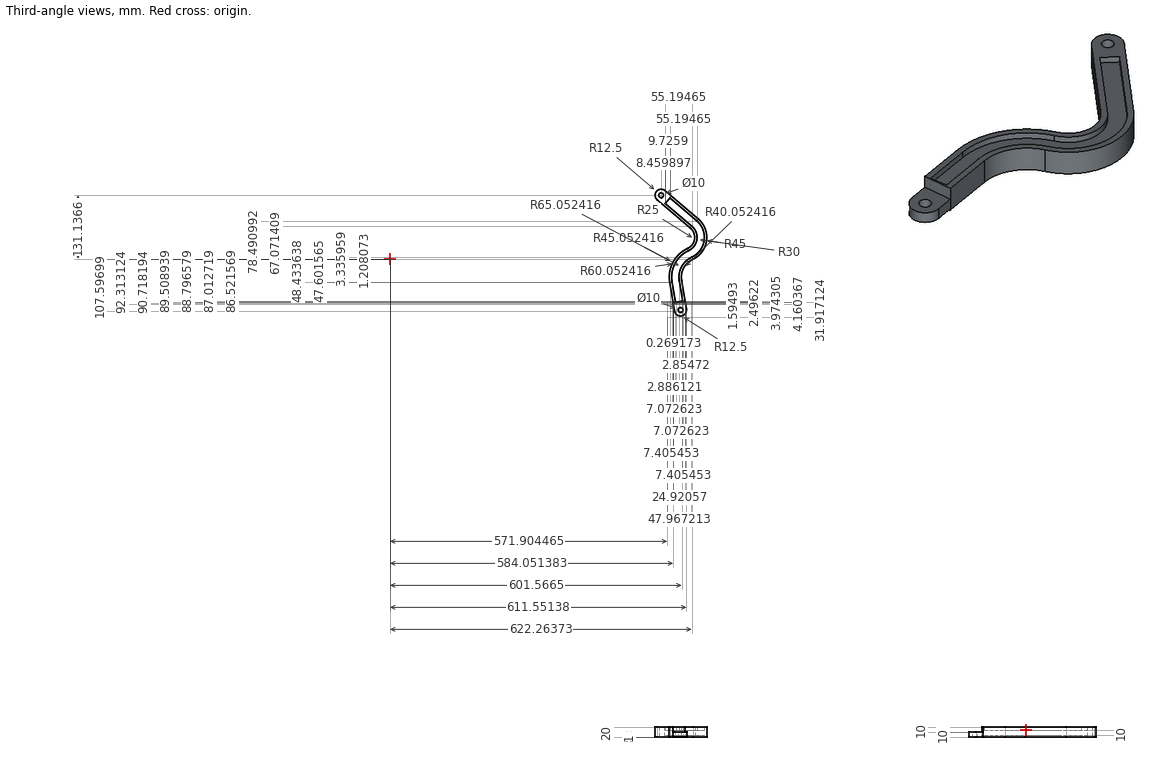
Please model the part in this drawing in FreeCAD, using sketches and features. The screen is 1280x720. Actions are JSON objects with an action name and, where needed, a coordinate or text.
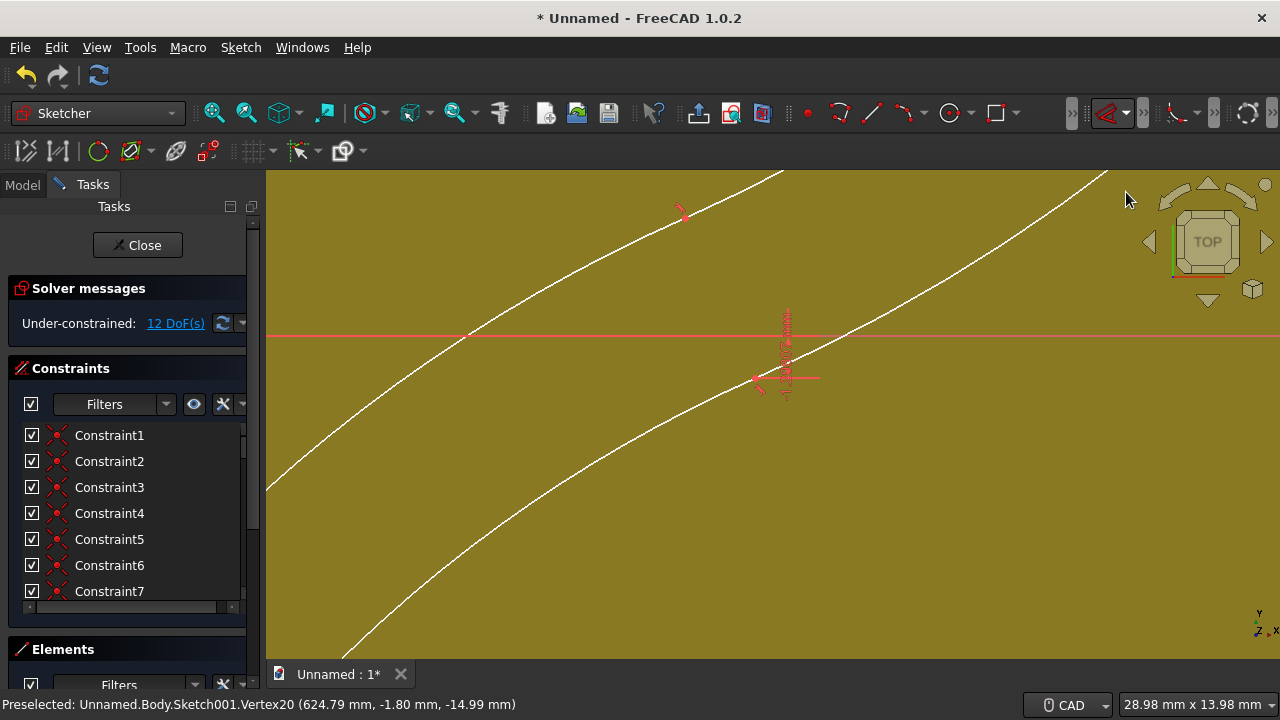
{"action": "scroll", "coordinate": [737, 454], "scroll_direction": "down", "scroll_amount": 16}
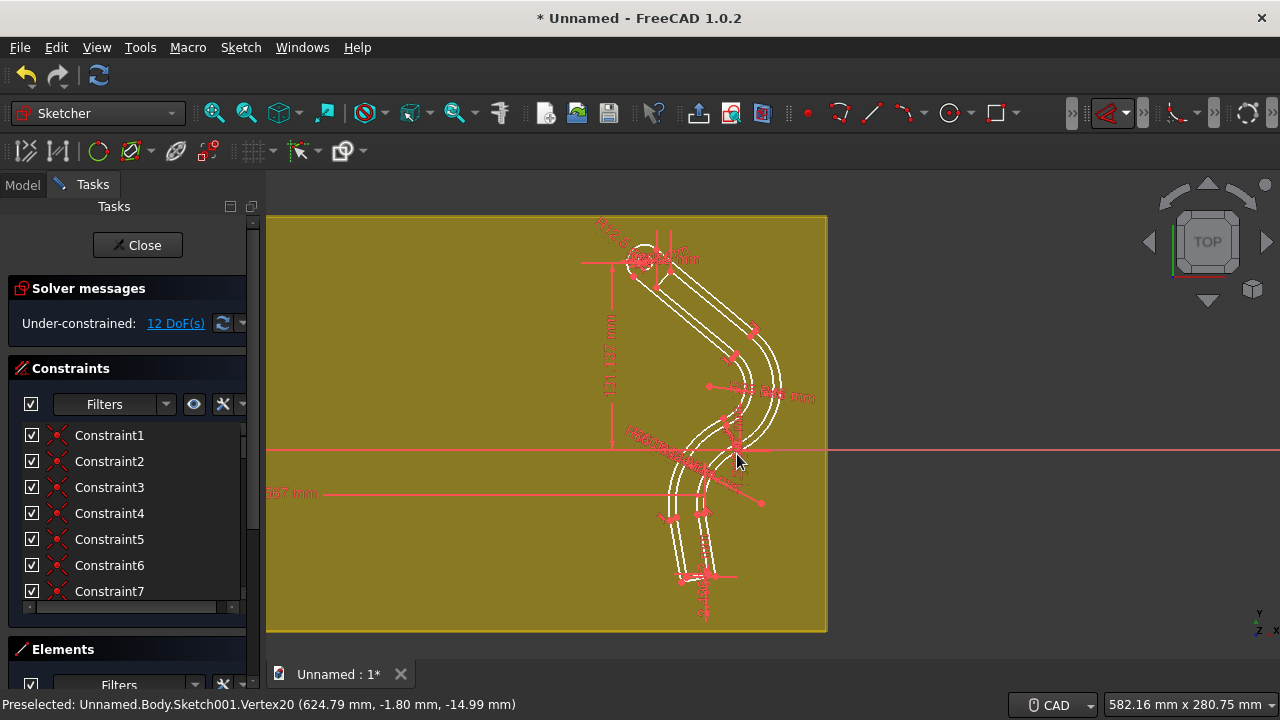
{"action": "scroll", "coordinate": [673, 539], "scroll_direction": "up", "scroll_amount": 7}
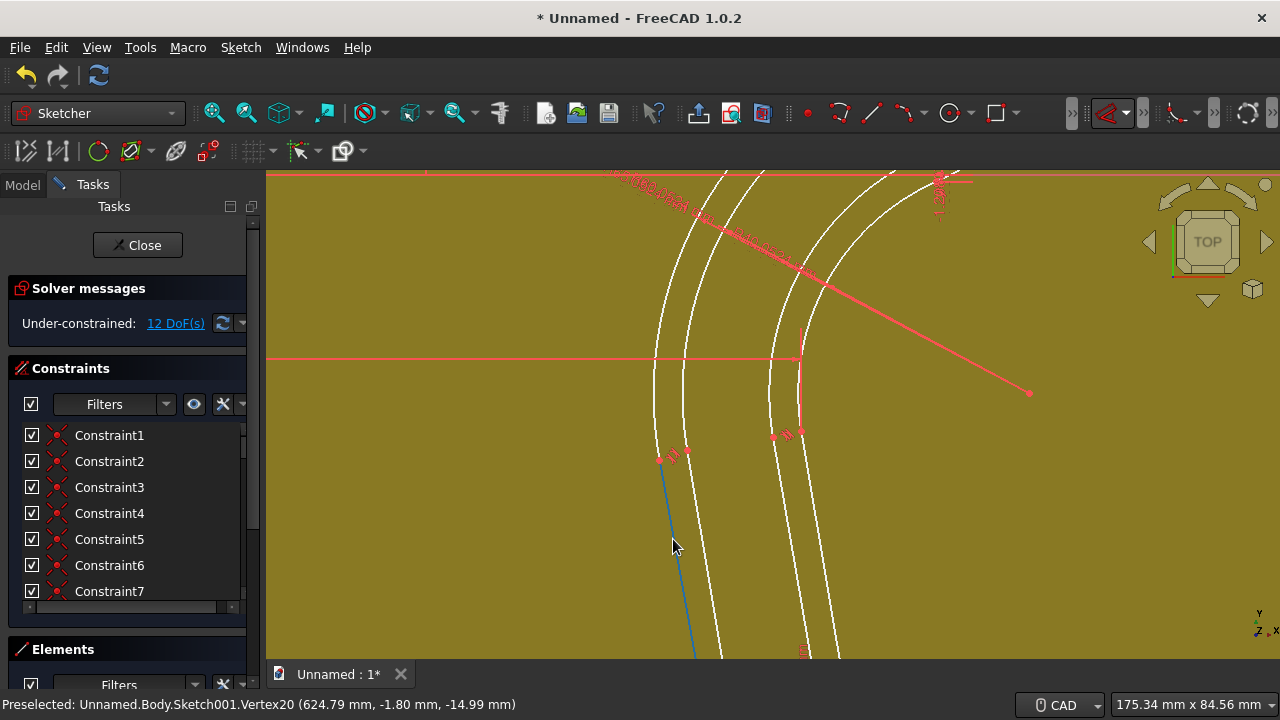
{"action": "left_click", "coordinate": [673, 536]}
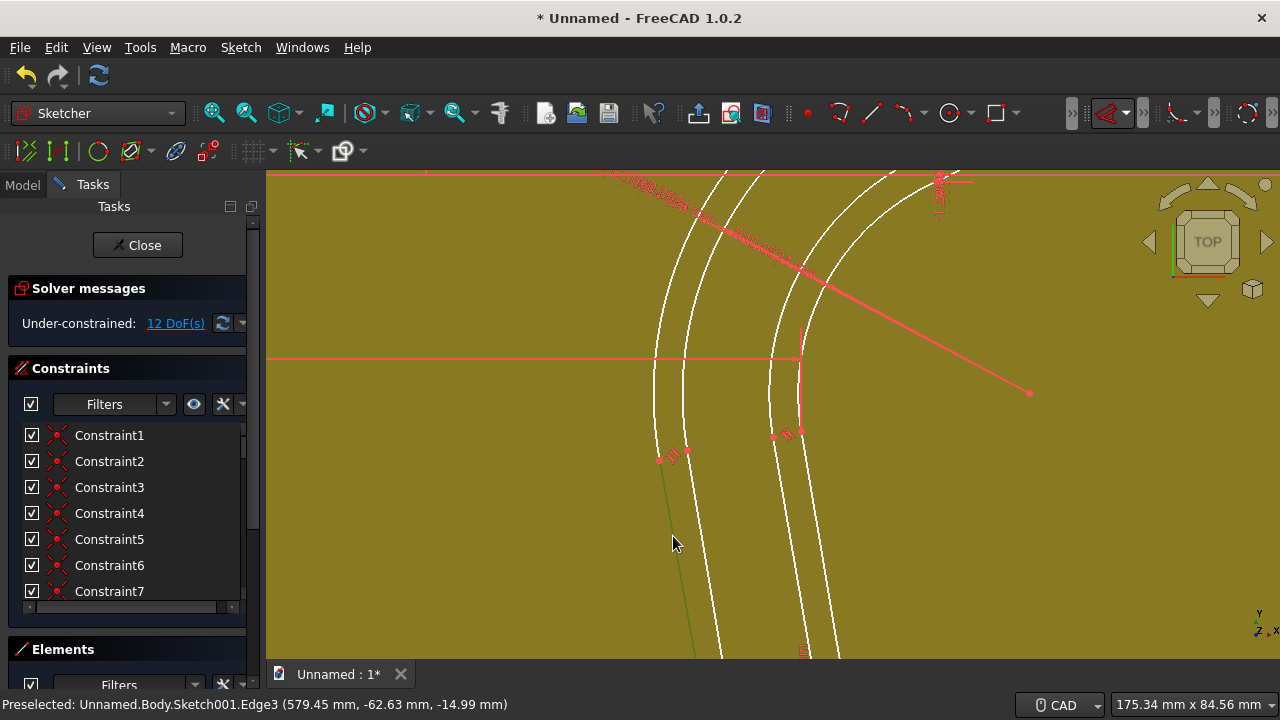
{"action": "left_click", "coordinate": [1128, 114]}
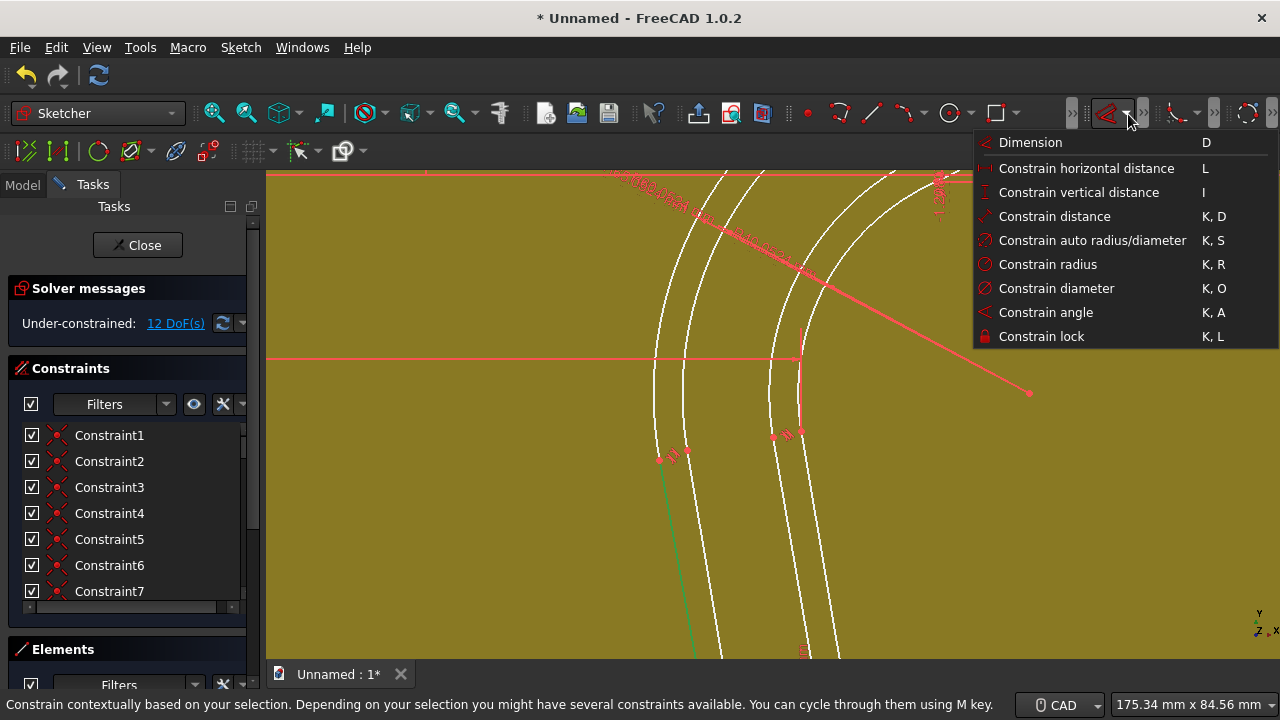
{"action": "left_click", "coordinate": [1126, 168]}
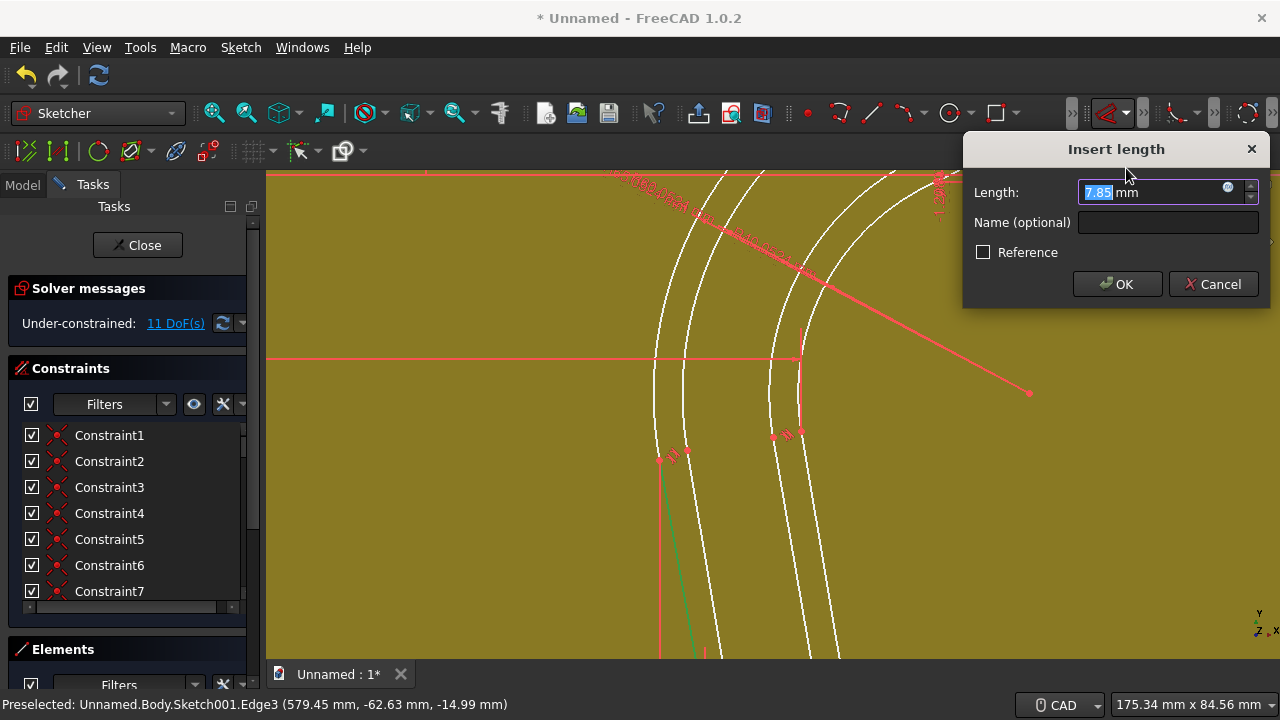
{"action": "type", "text": "7.405453"}
{"action": "key", "text": "Return"}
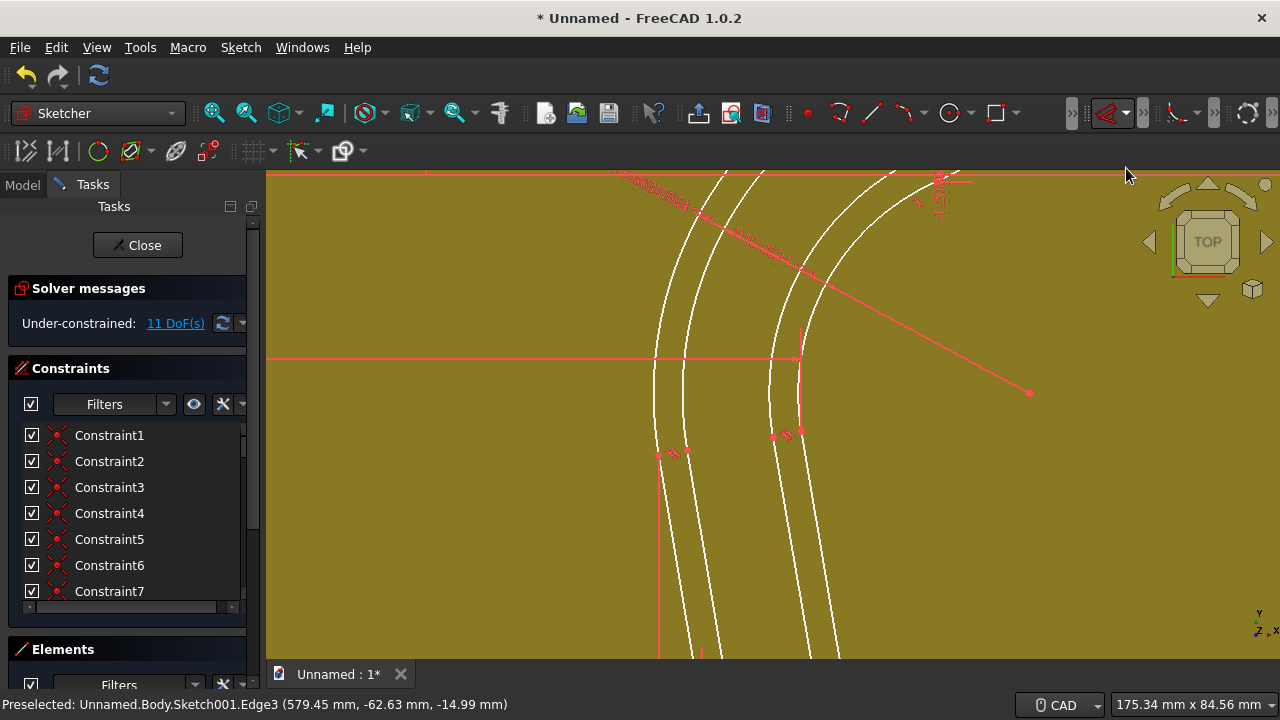
{"action": "scroll", "coordinate": [673, 539], "scroll_direction": "down", "scroll_amount": 7}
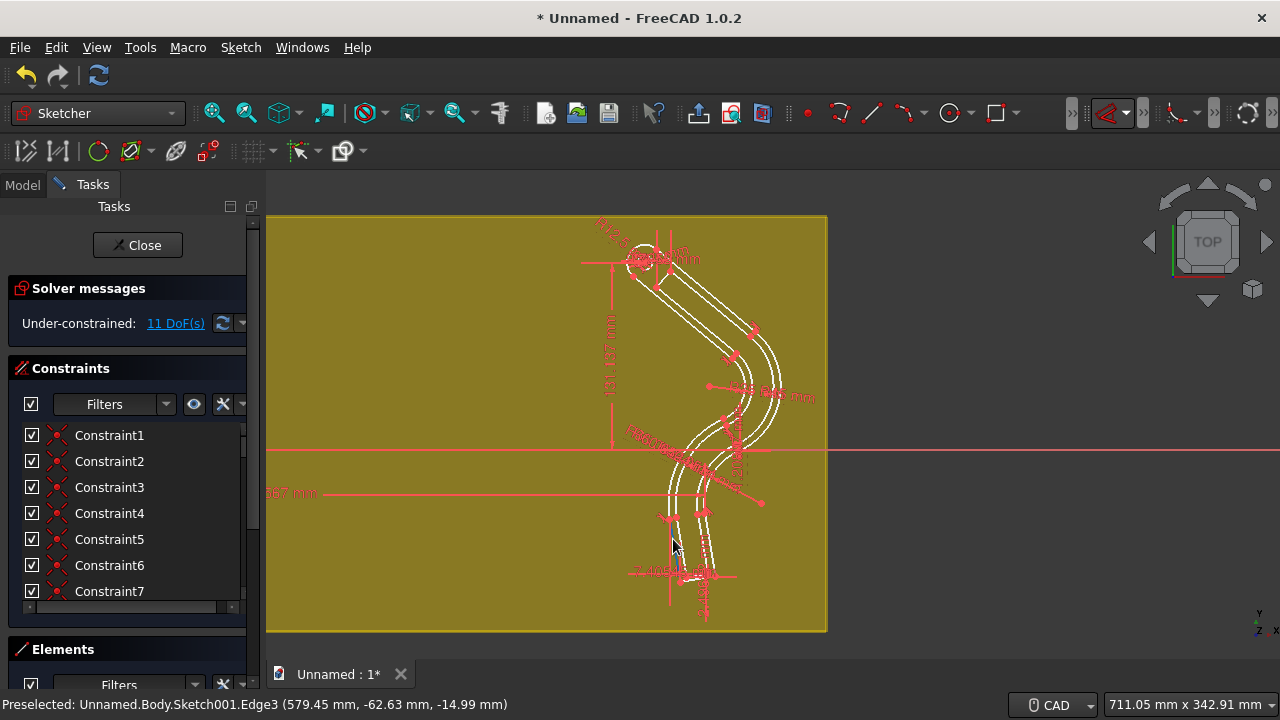
{"action": "scroll", "coordinate": [691, 580], "scroll_direction": "up", "scroll_amount": 10}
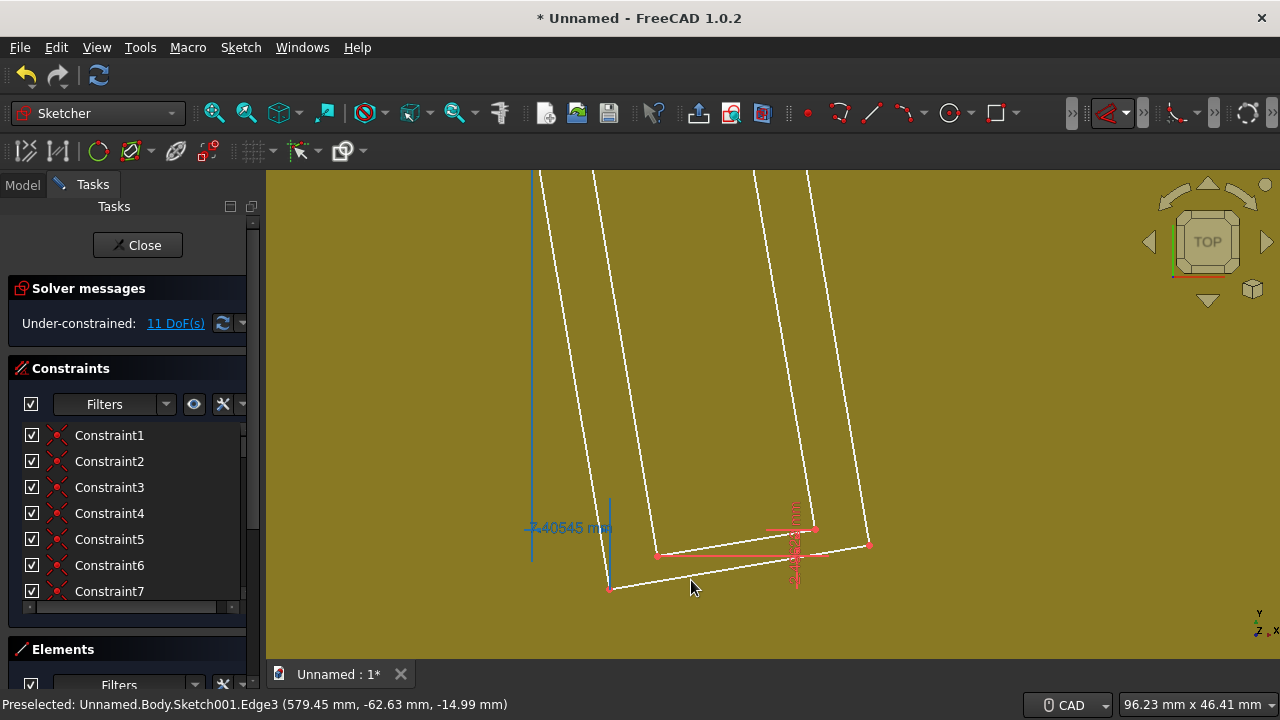
{"action": "left_click", "coordinate": [688, 576]}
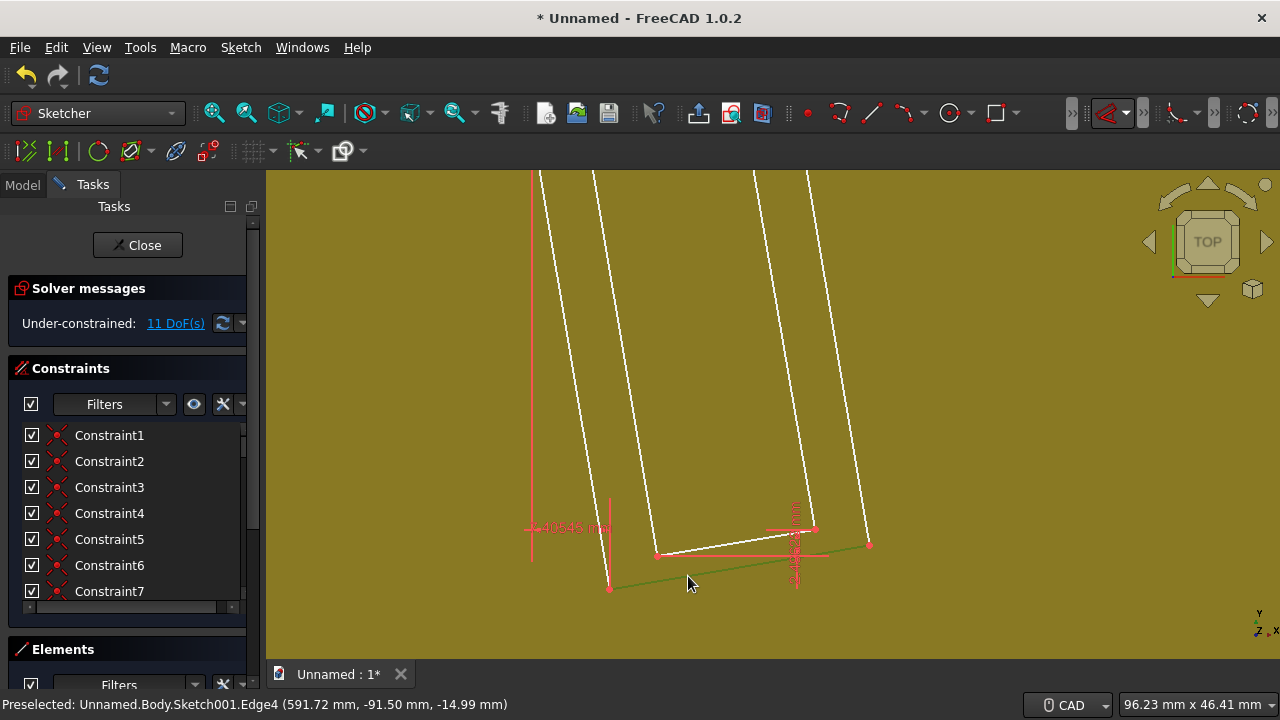
{"action": "left_click", "coordinate": [1128, 114]}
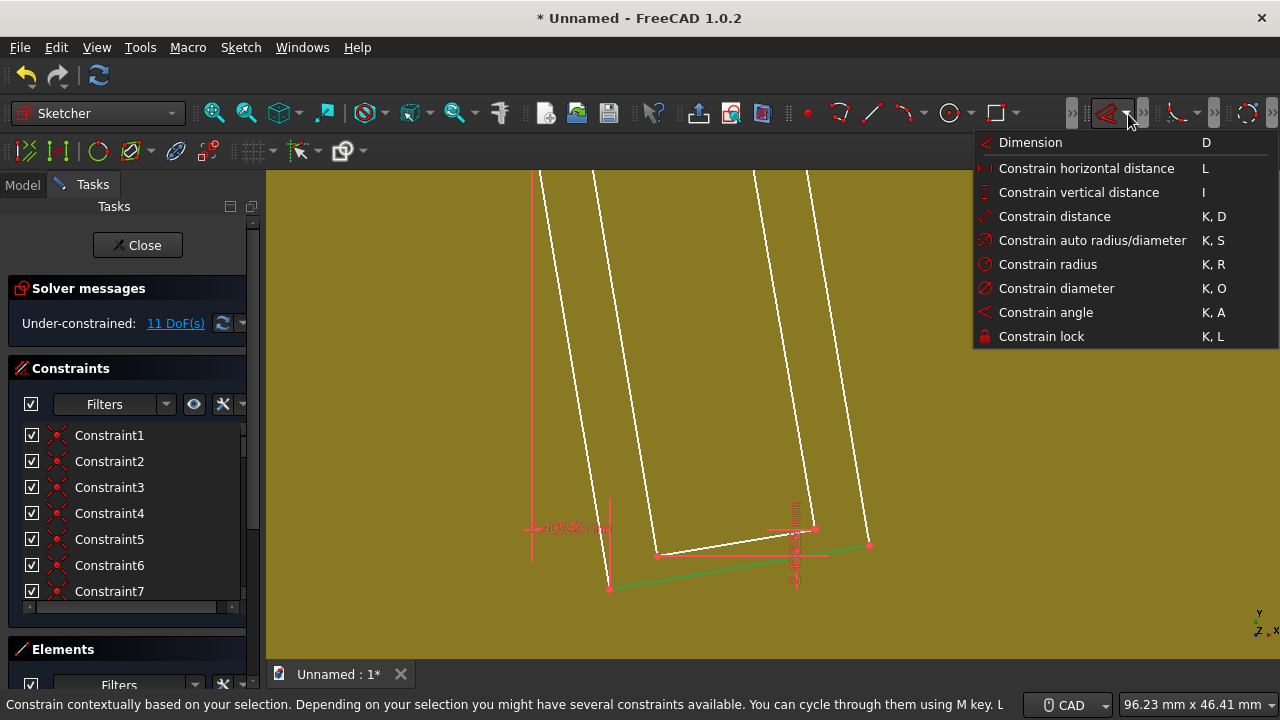
{"action": "left_click", "coordinate": [1126, 192]}